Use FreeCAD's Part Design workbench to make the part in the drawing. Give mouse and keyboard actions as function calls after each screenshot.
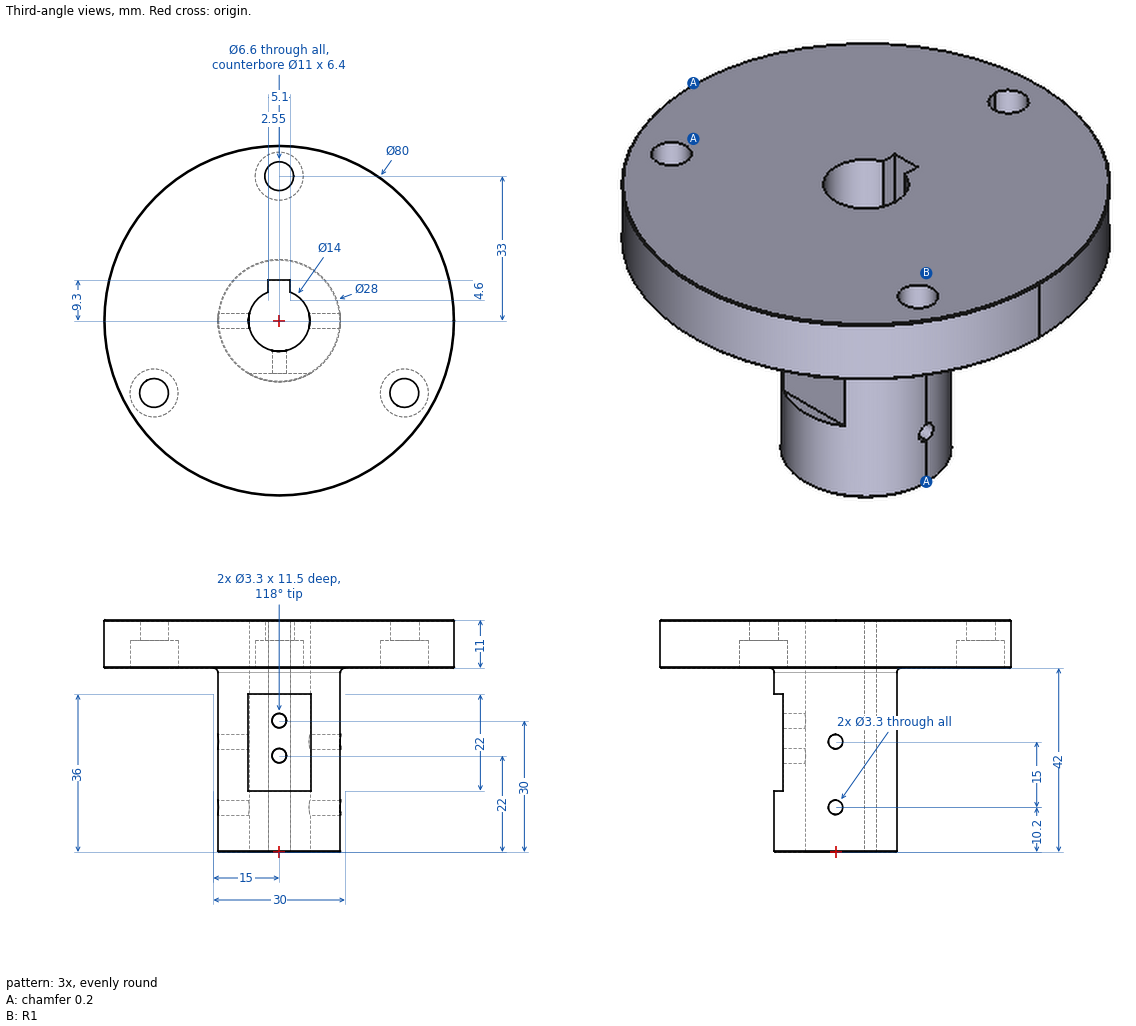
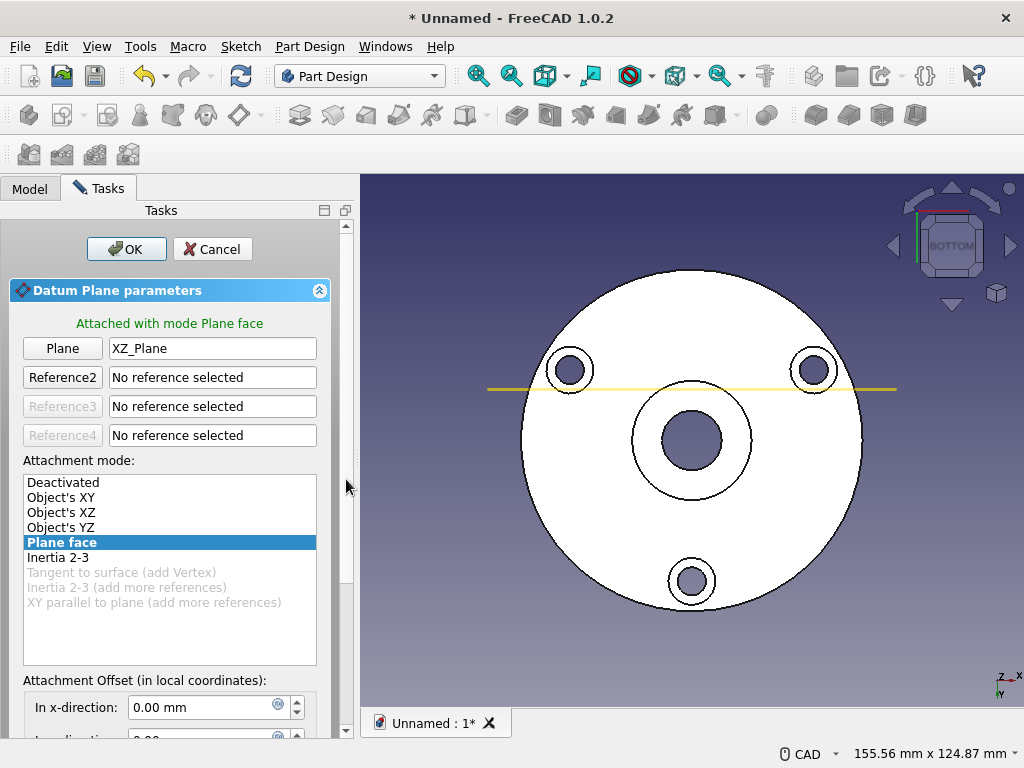
click(127, 249)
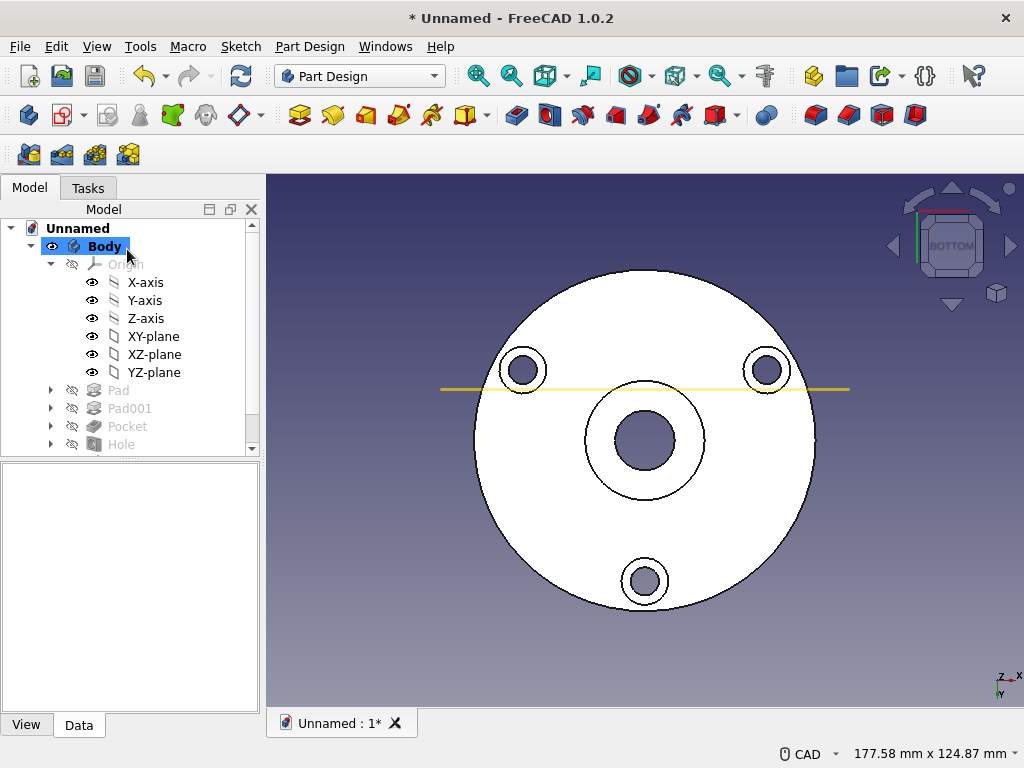
scroll(101, 332, down, 3)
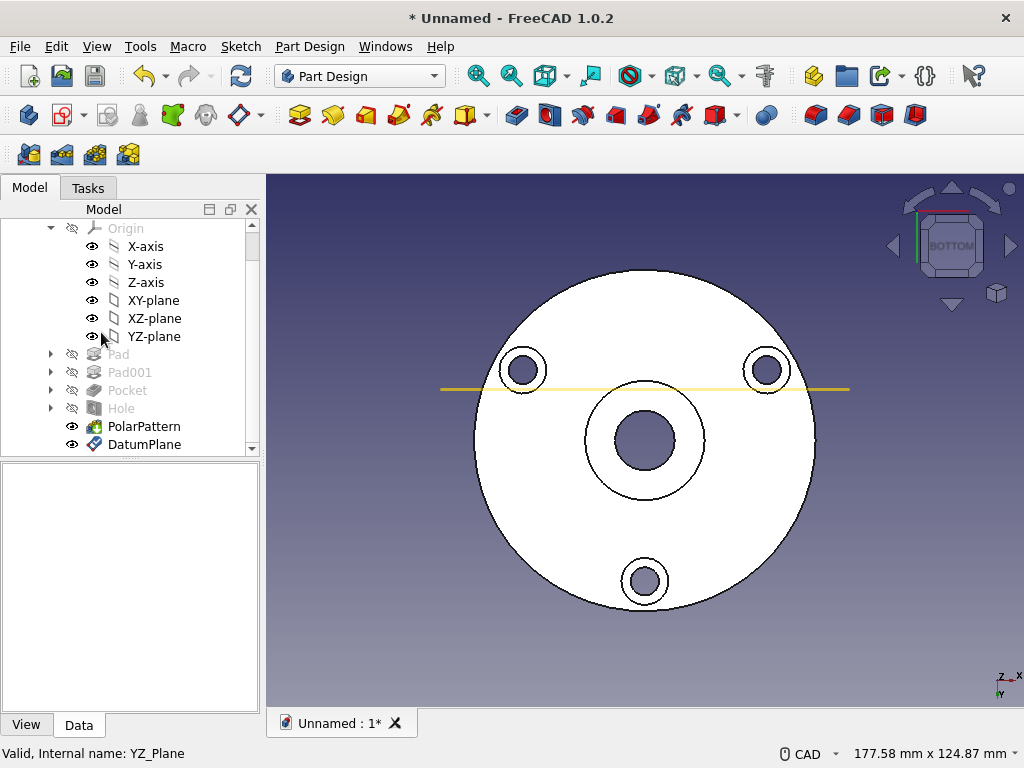
click(117, 444)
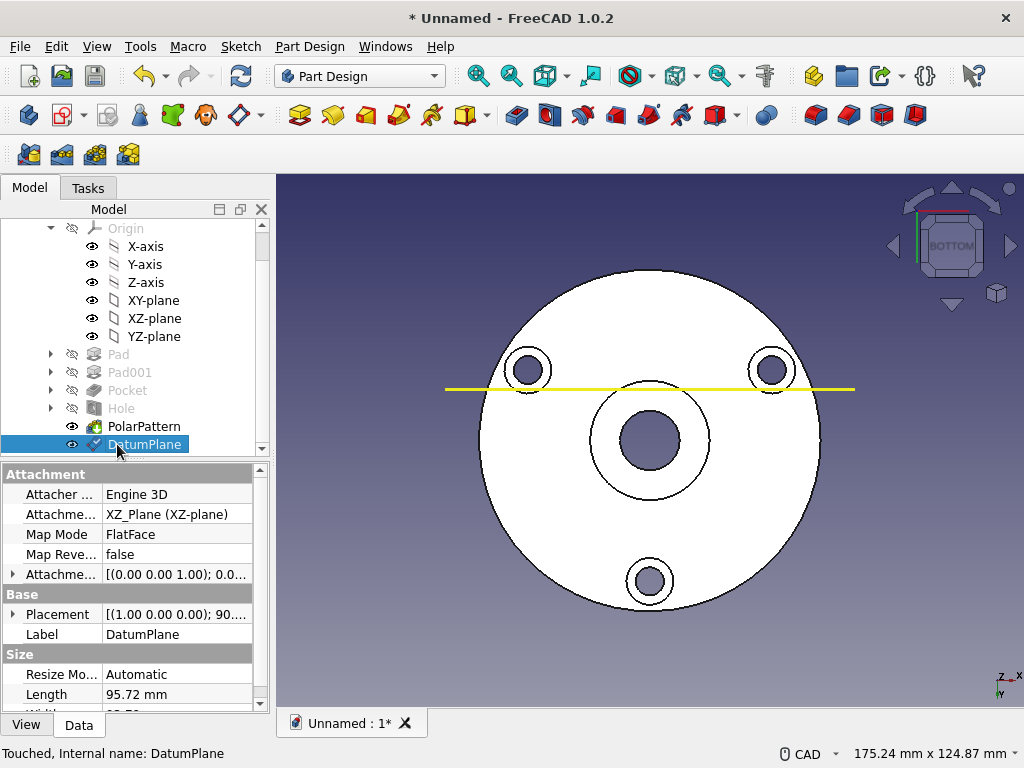
click(62, 116)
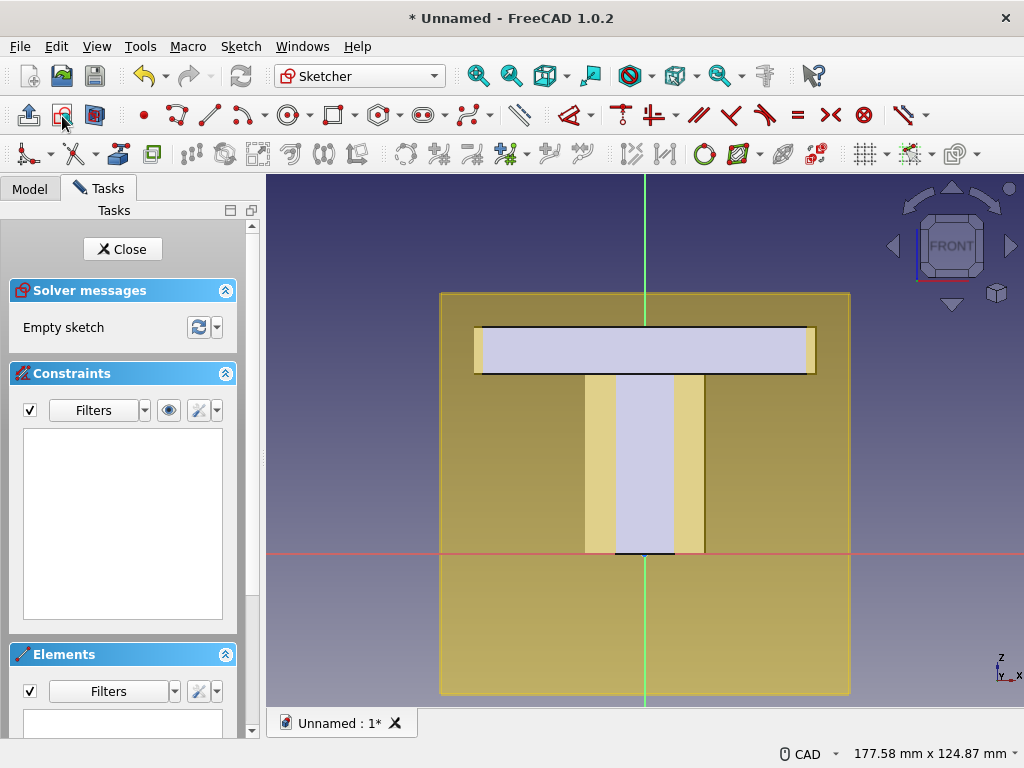
key(q)
key(s)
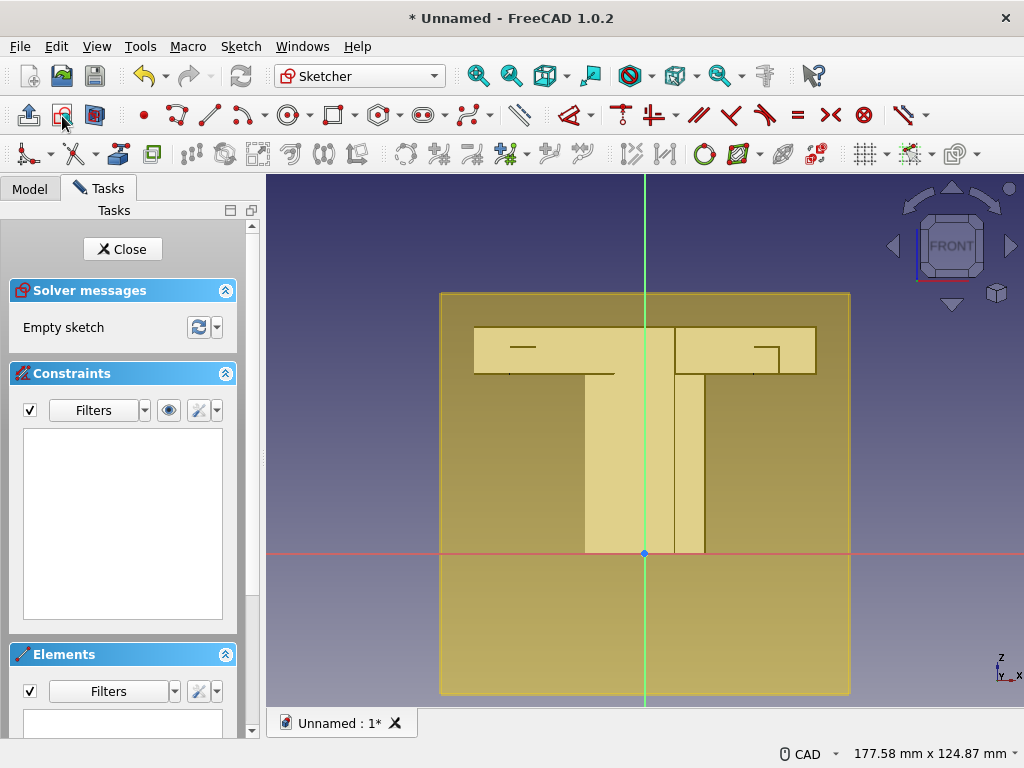
scroll(701, 506, up, 4)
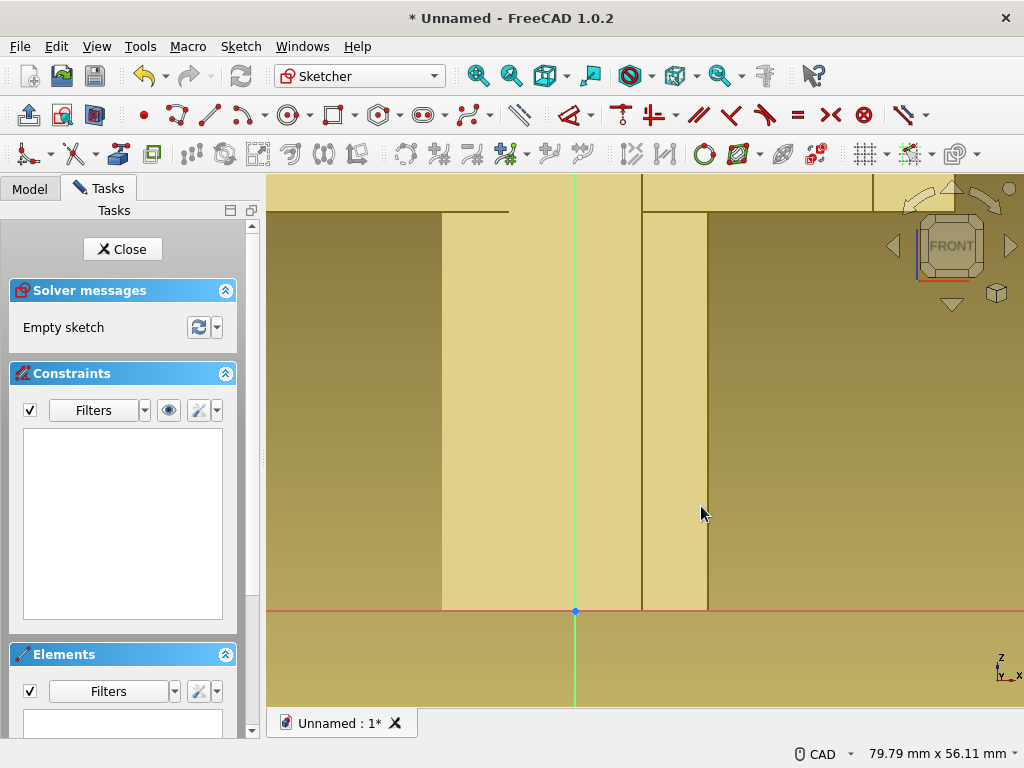
key(g)
key(r)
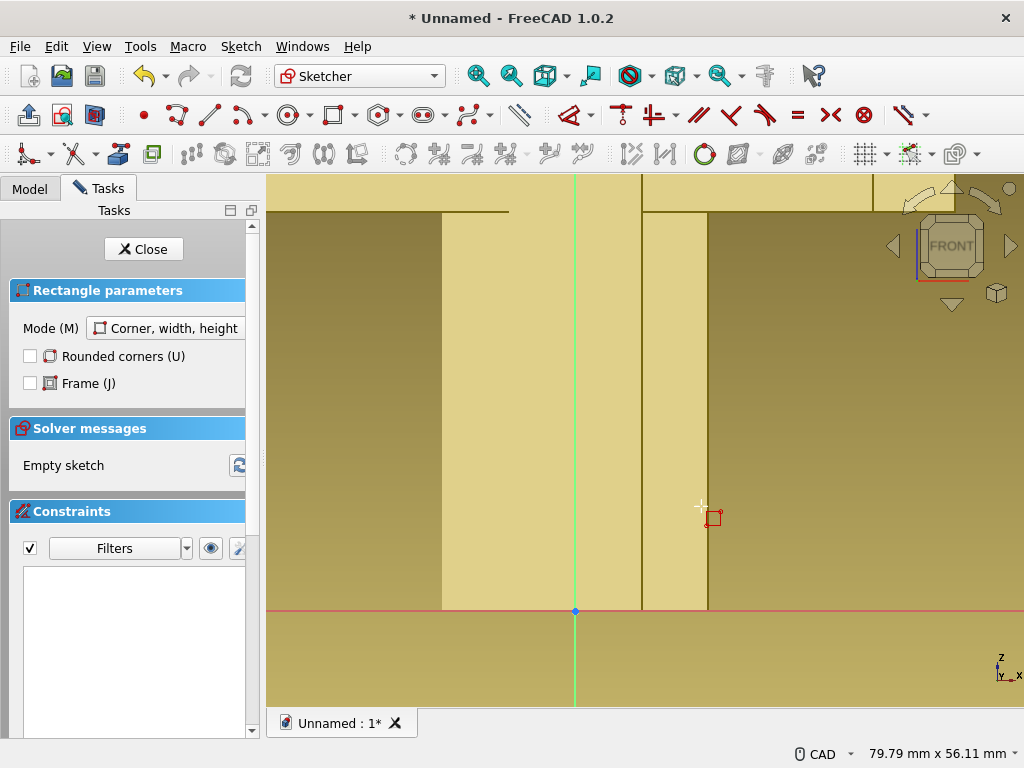
click(433, 269)
move(718, 478)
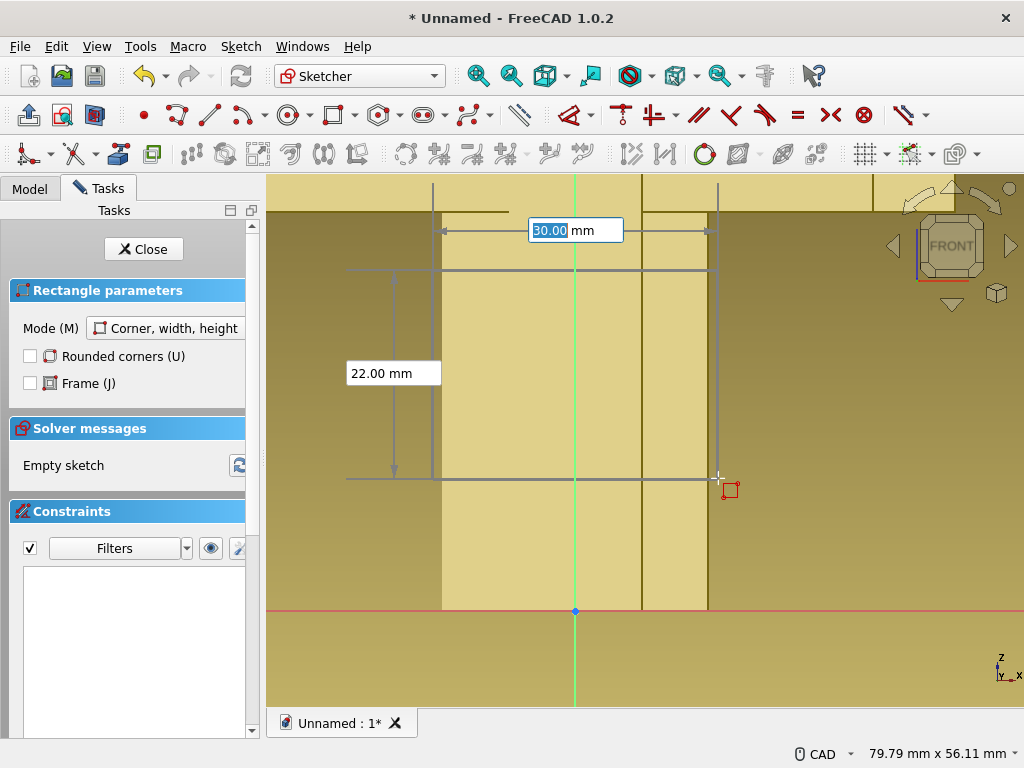
text(30)
key(Tab)
text(22)
key(Return)
key(Escape)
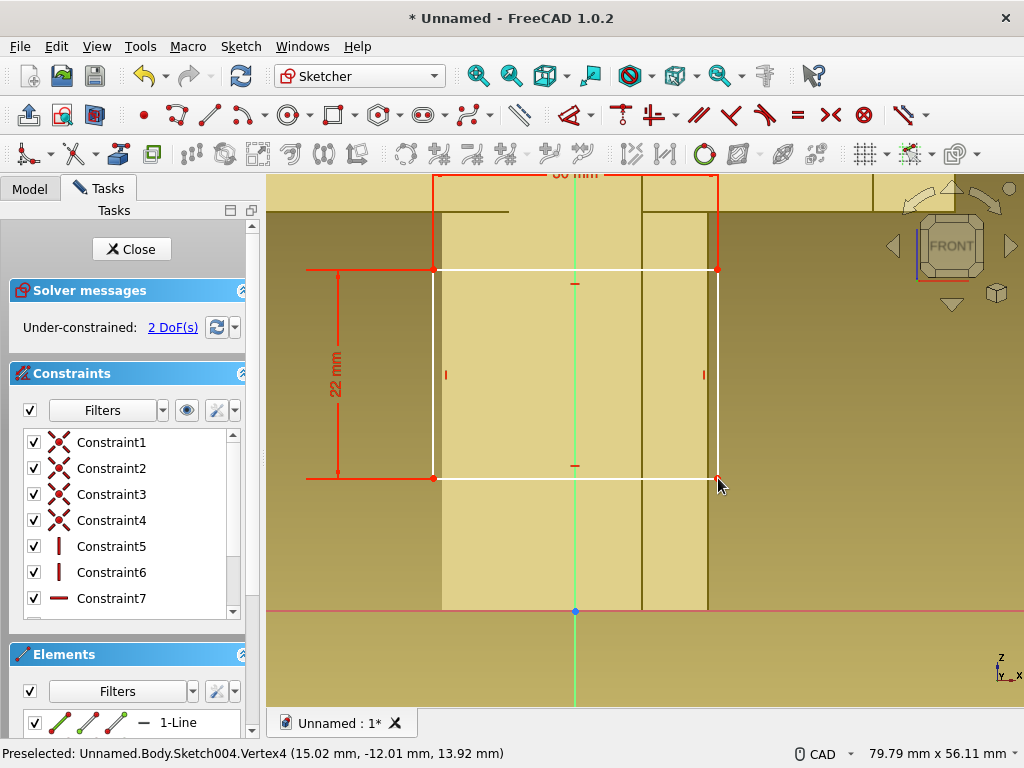
click(433, 270)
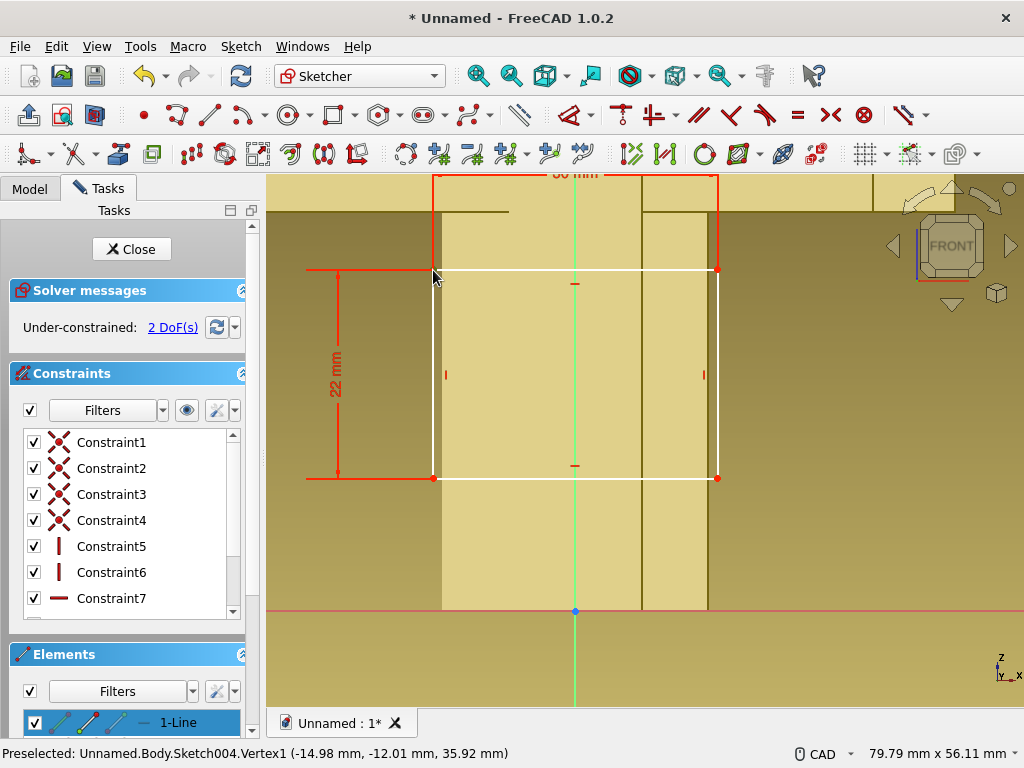
click(590, 116)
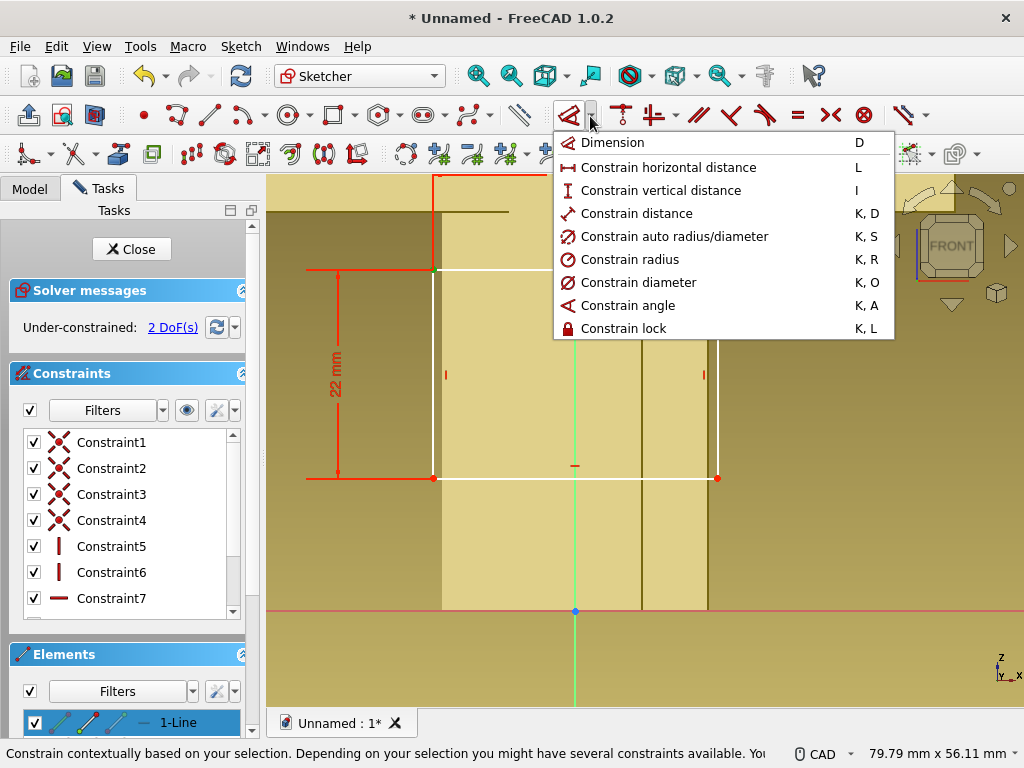
click(724, 168)